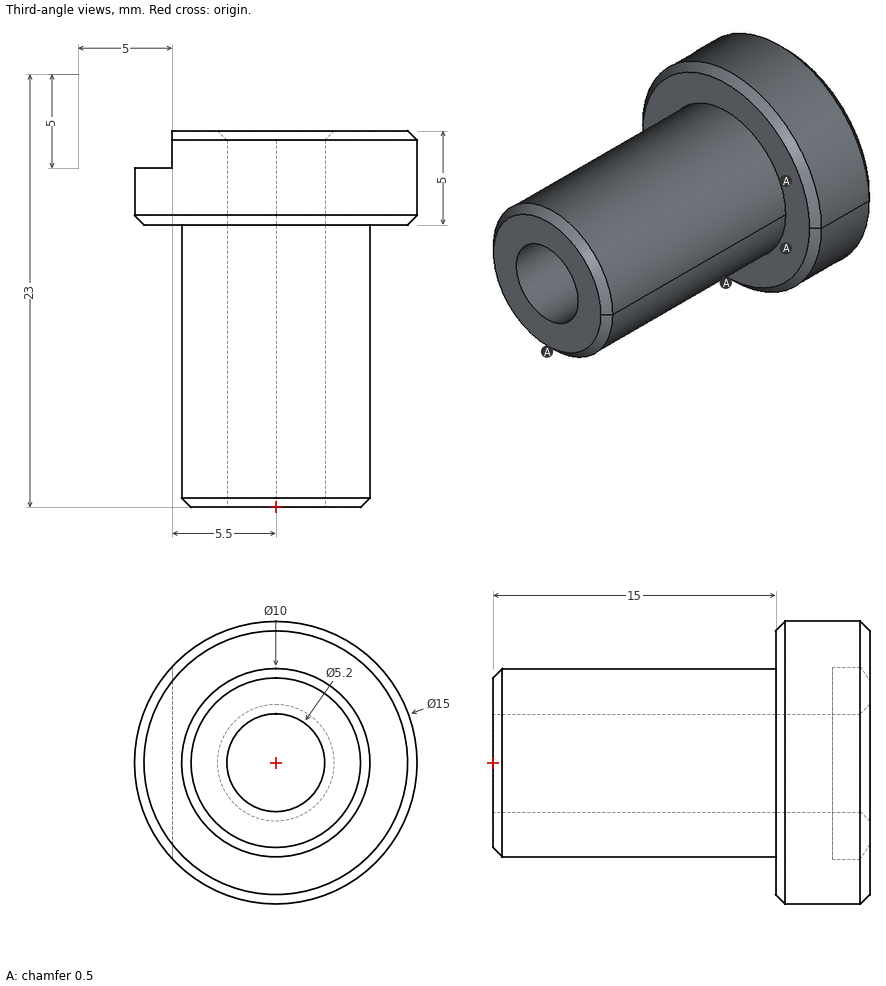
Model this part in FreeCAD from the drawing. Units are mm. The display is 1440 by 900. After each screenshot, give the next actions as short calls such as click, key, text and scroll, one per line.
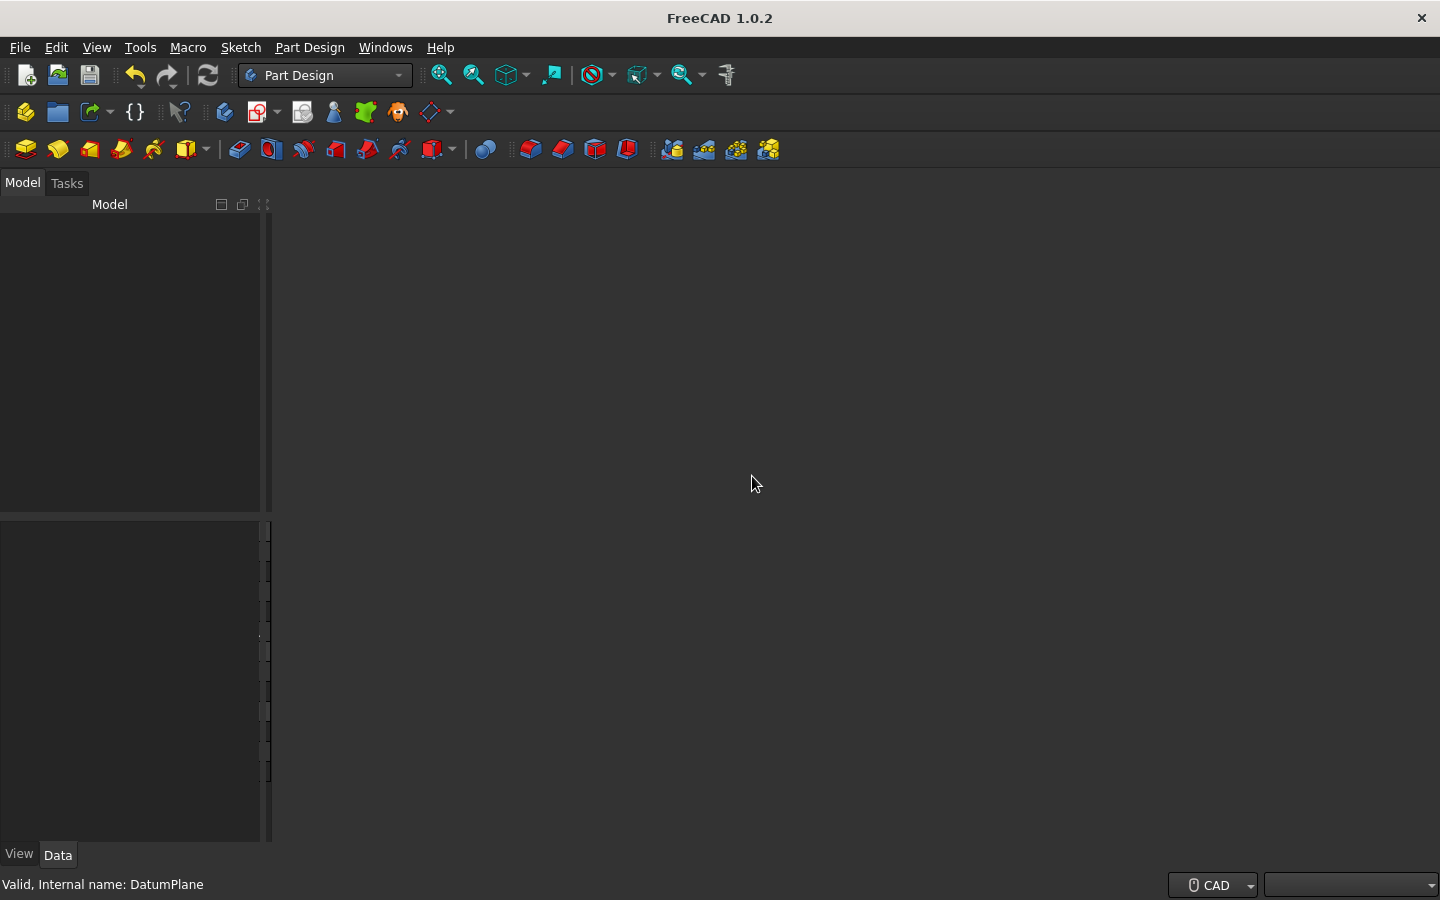
click(26, 76)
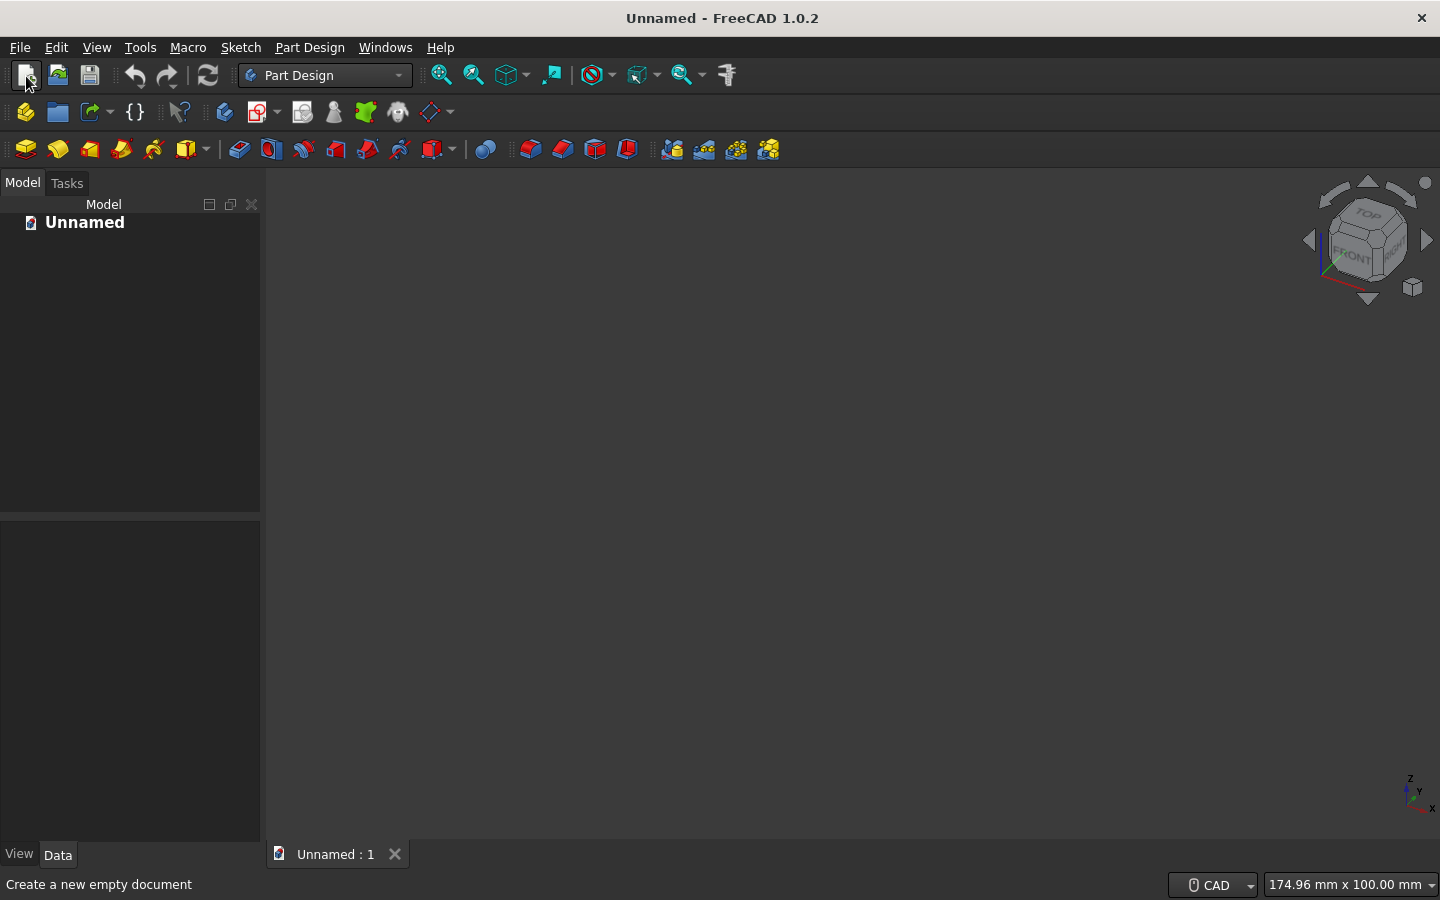
click(258, 112)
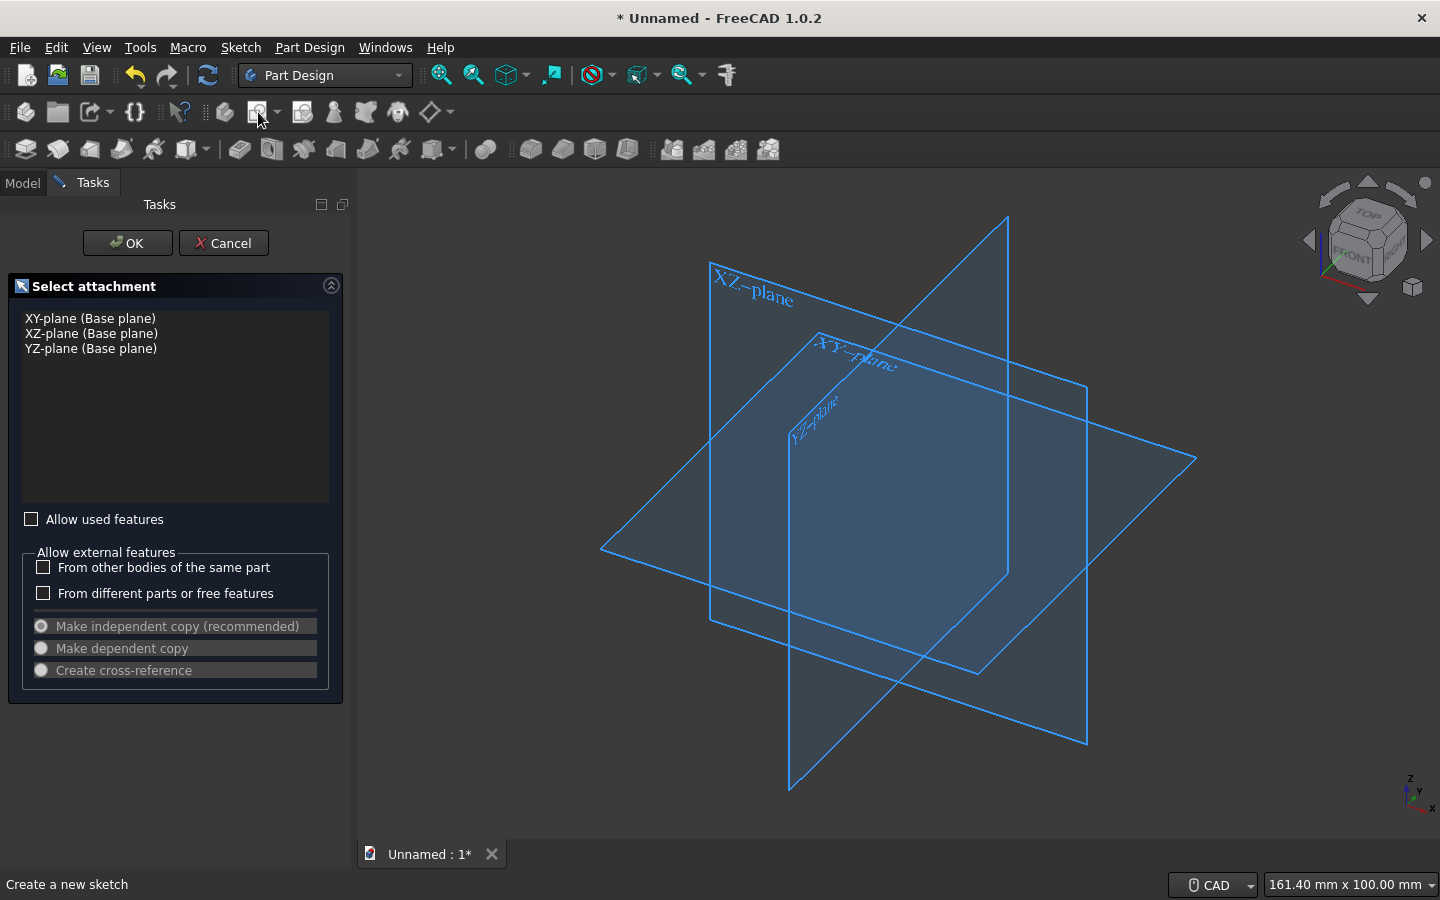
click(82, 334)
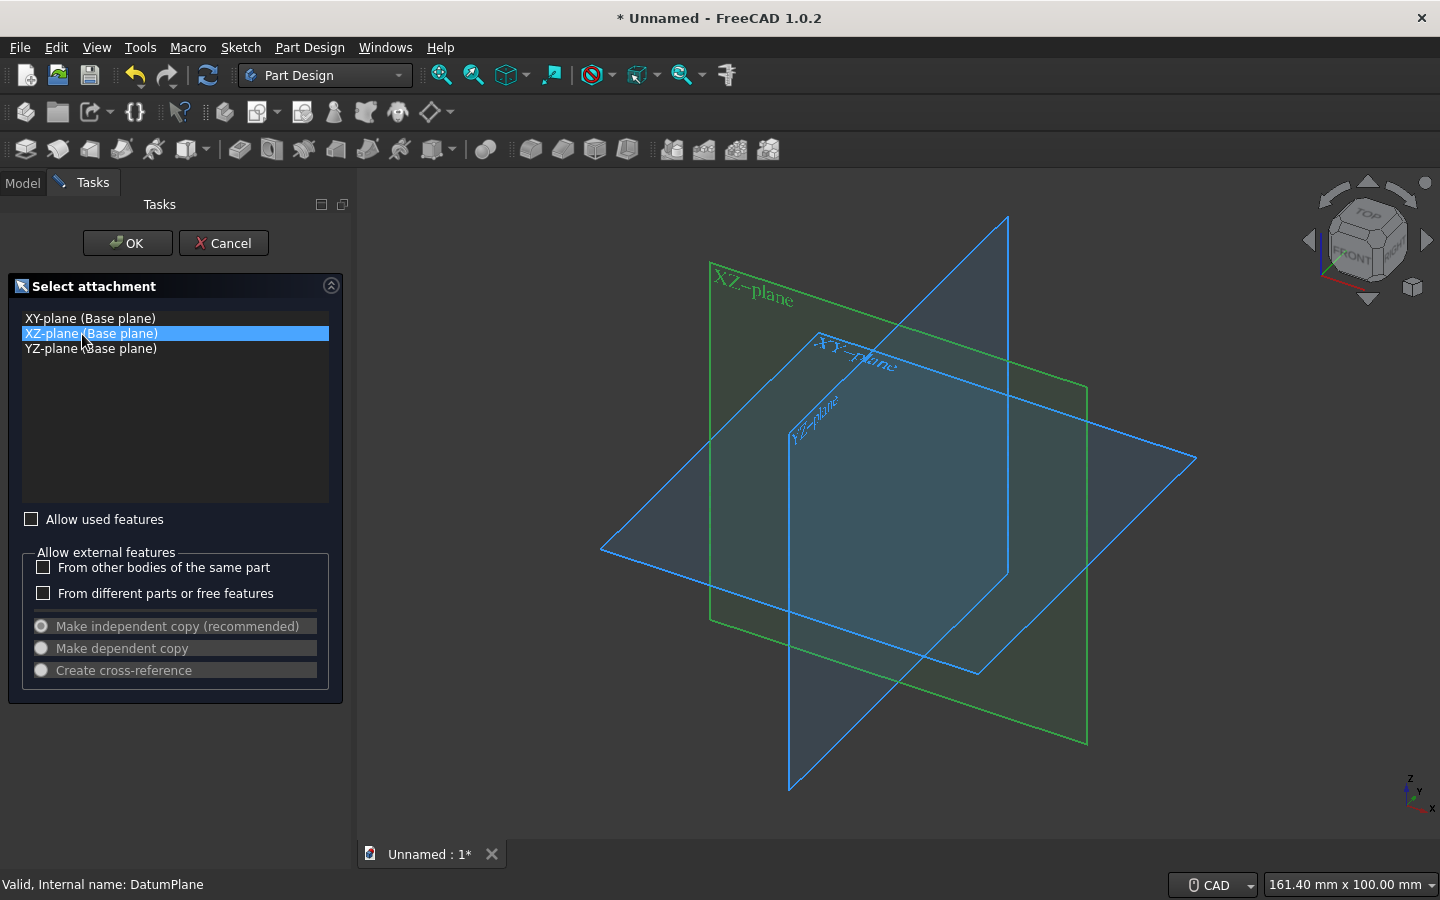
click(128, 243)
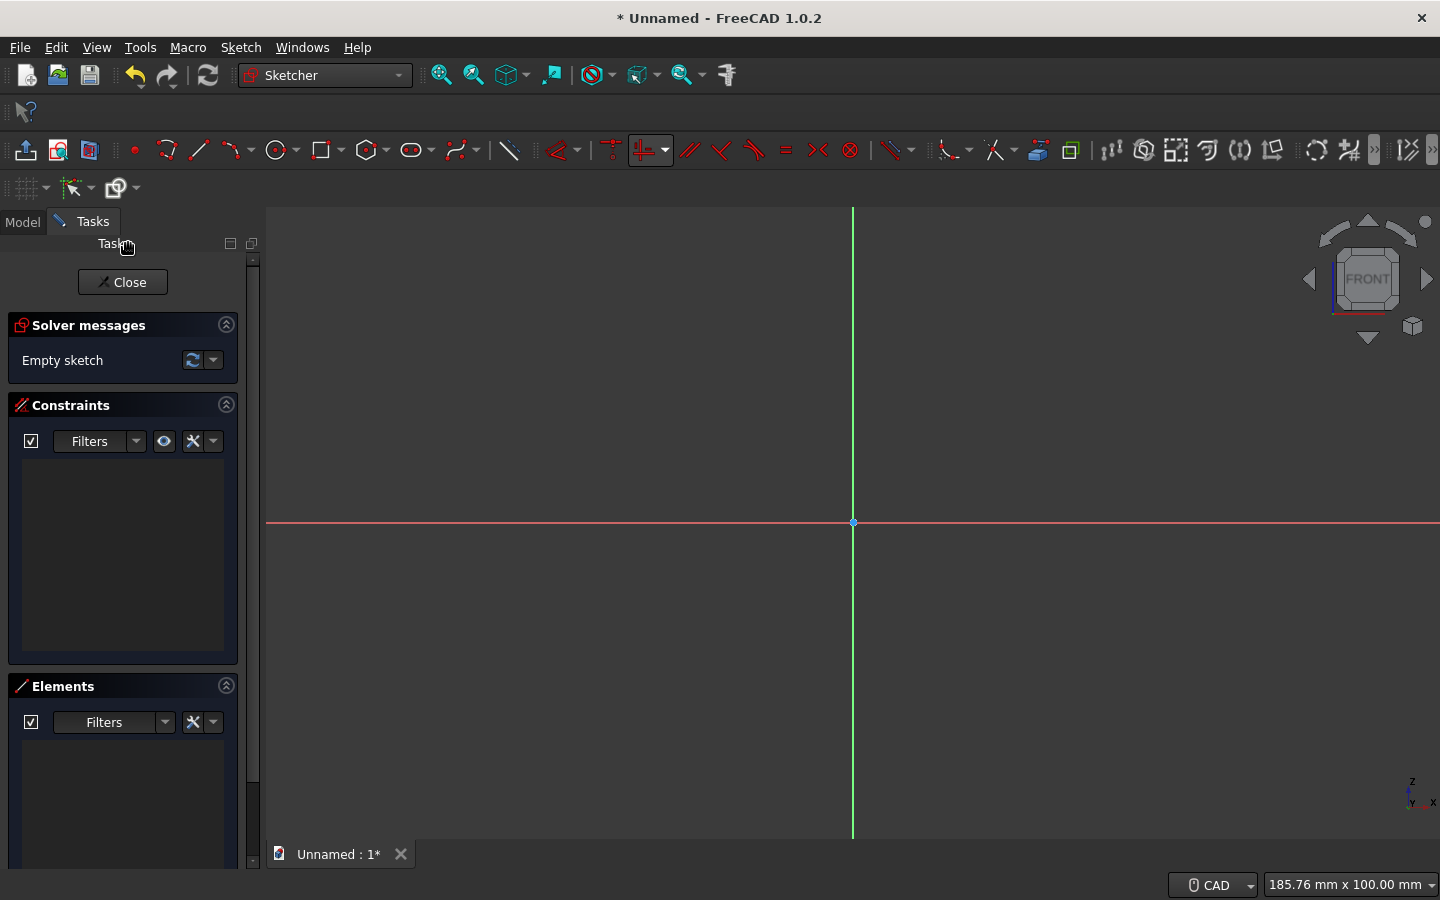
scroll(867, 523, up, 9)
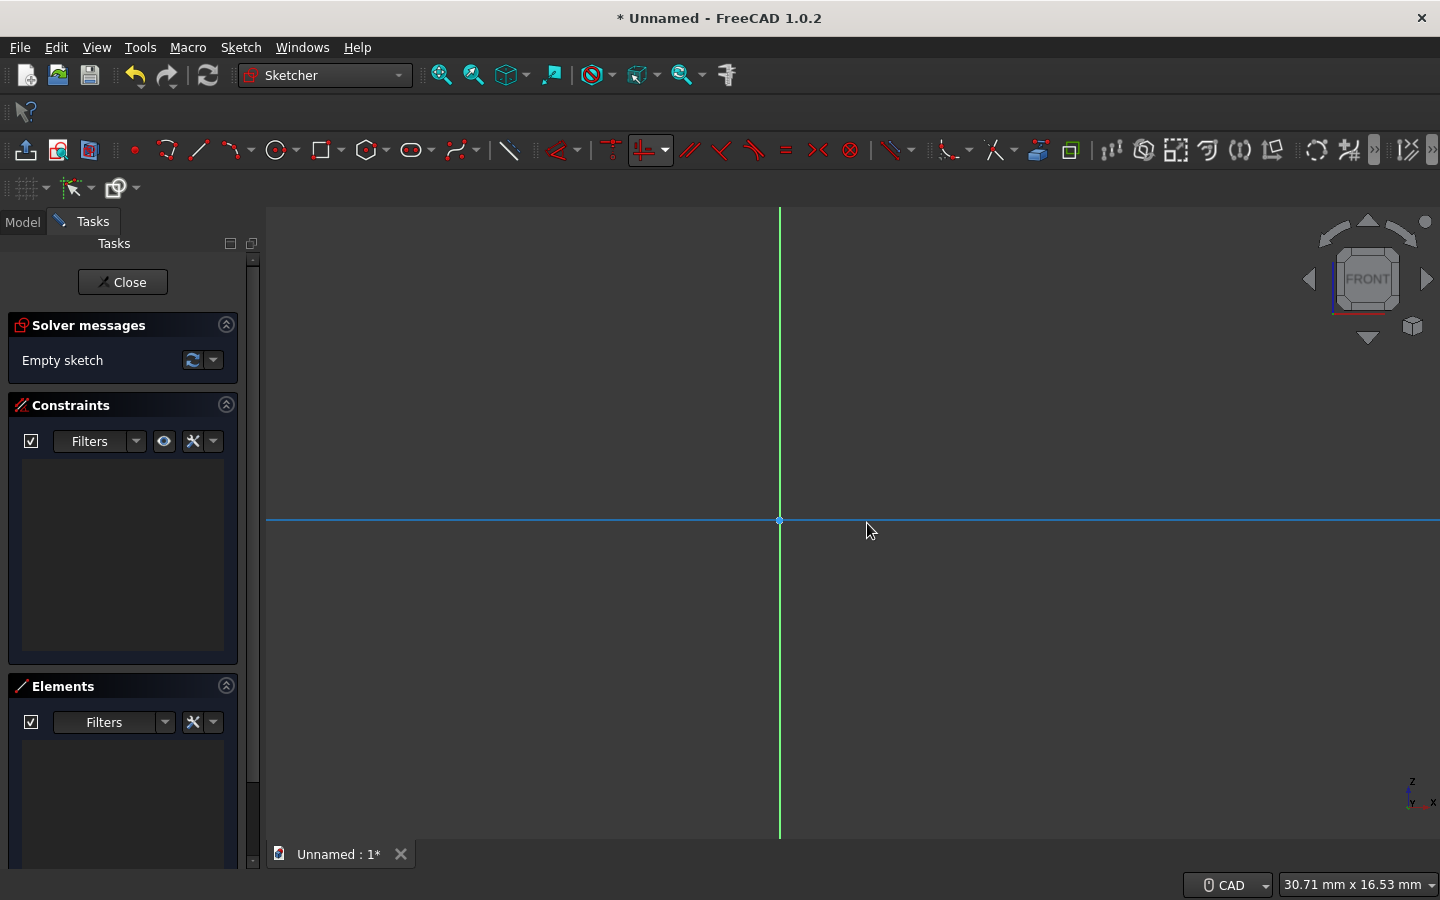
click(276, 150)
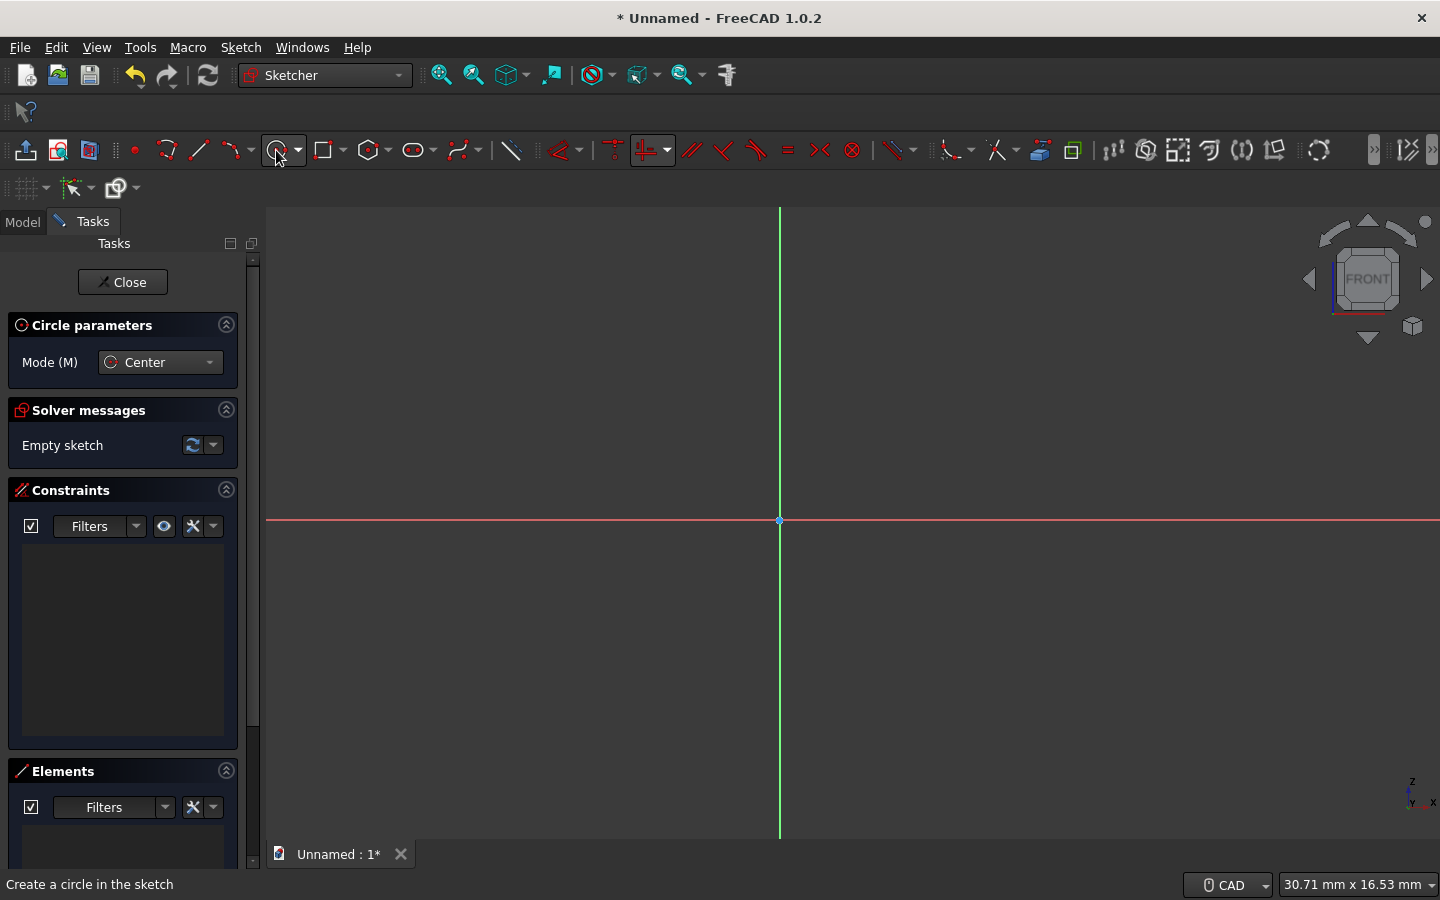
click(780, 520)
click(915, 385)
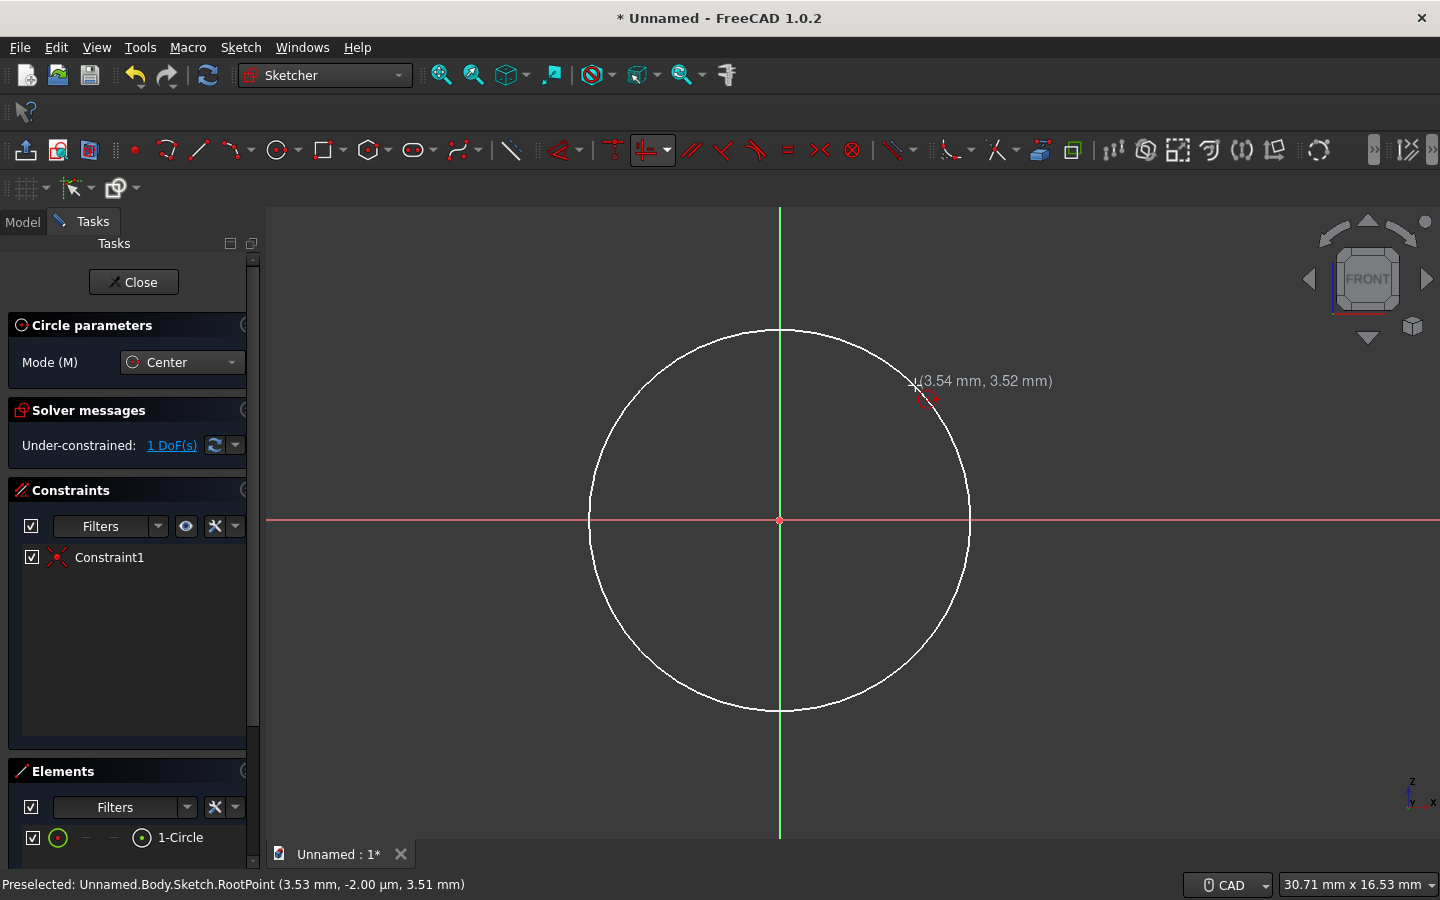
click(780, 520)
click(850, 450)
key(Escape)